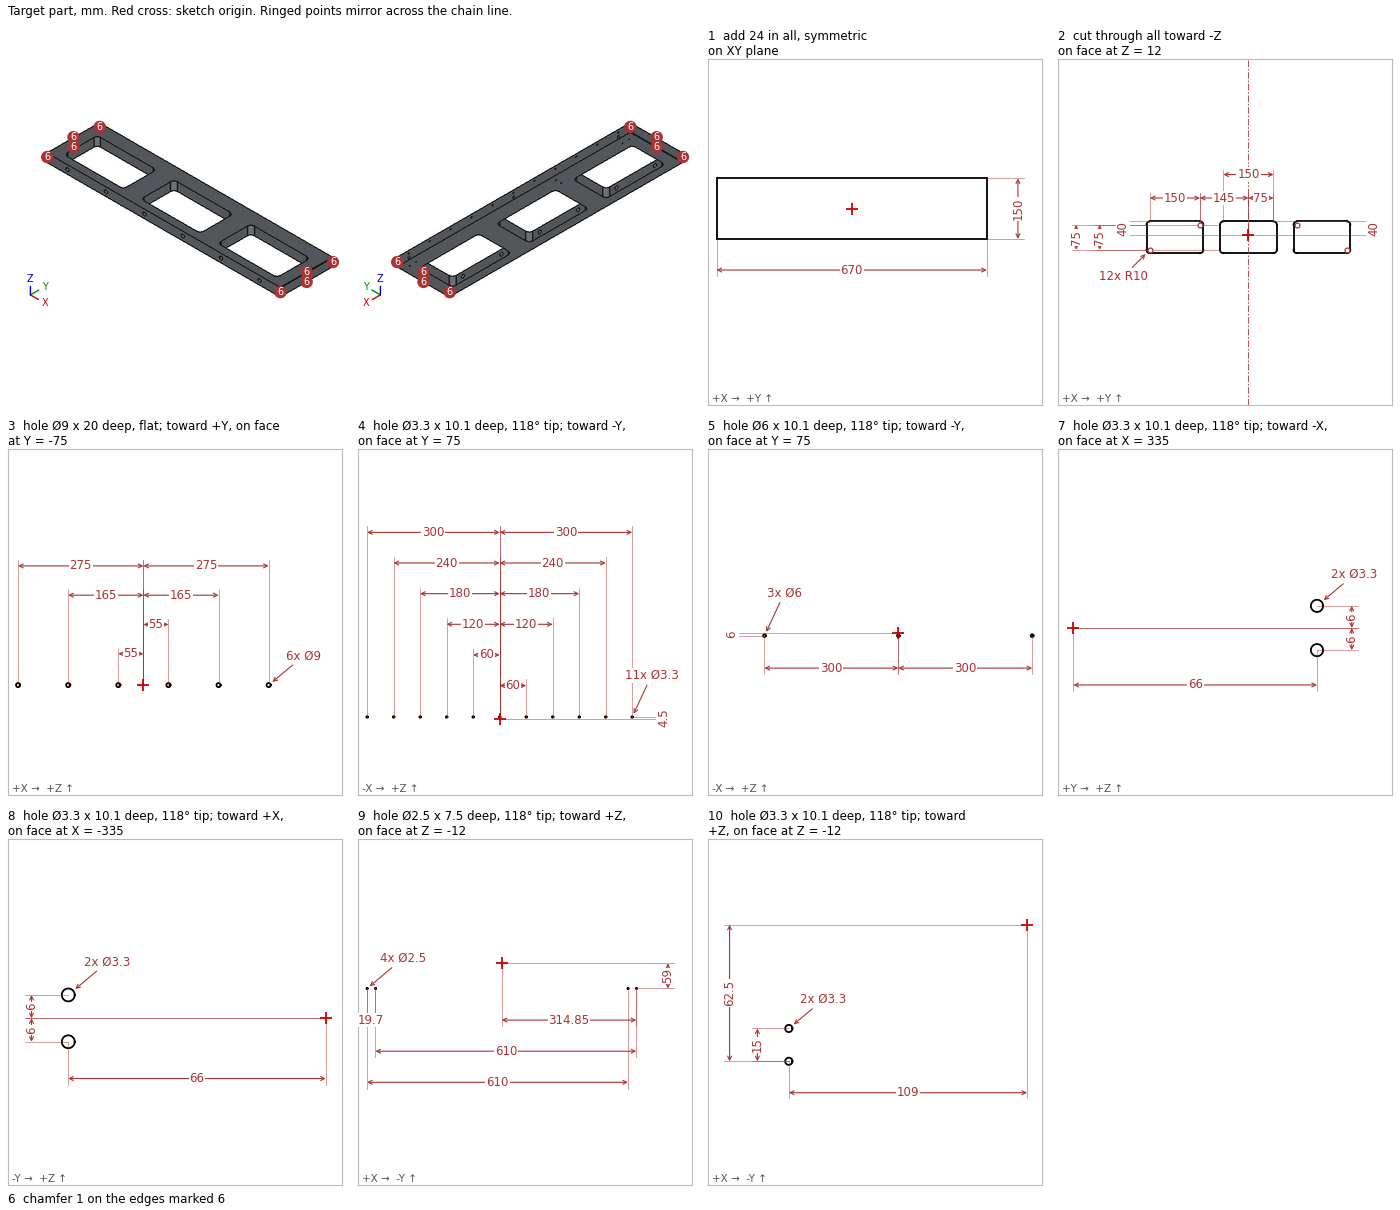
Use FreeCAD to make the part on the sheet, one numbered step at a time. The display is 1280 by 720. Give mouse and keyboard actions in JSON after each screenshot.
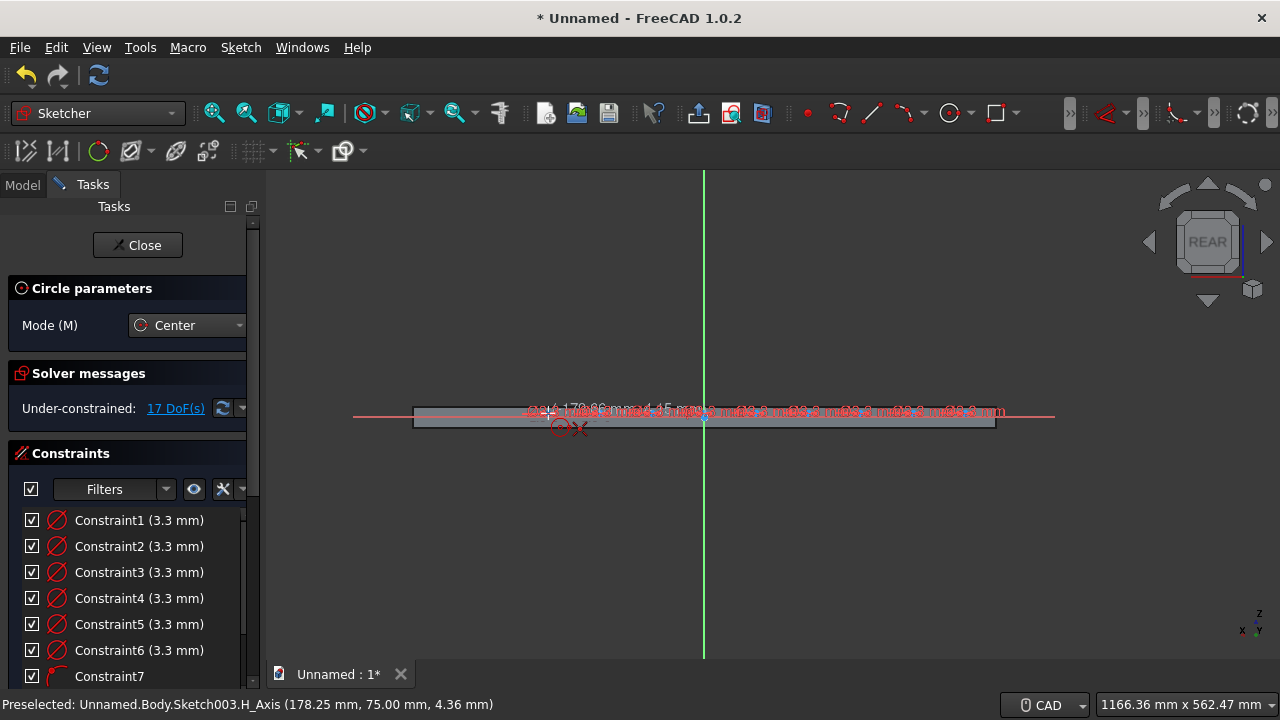
{"action": "scroll", "coordinate": [496, 413], "scroll_direction": "up", "scroll_amount": 14}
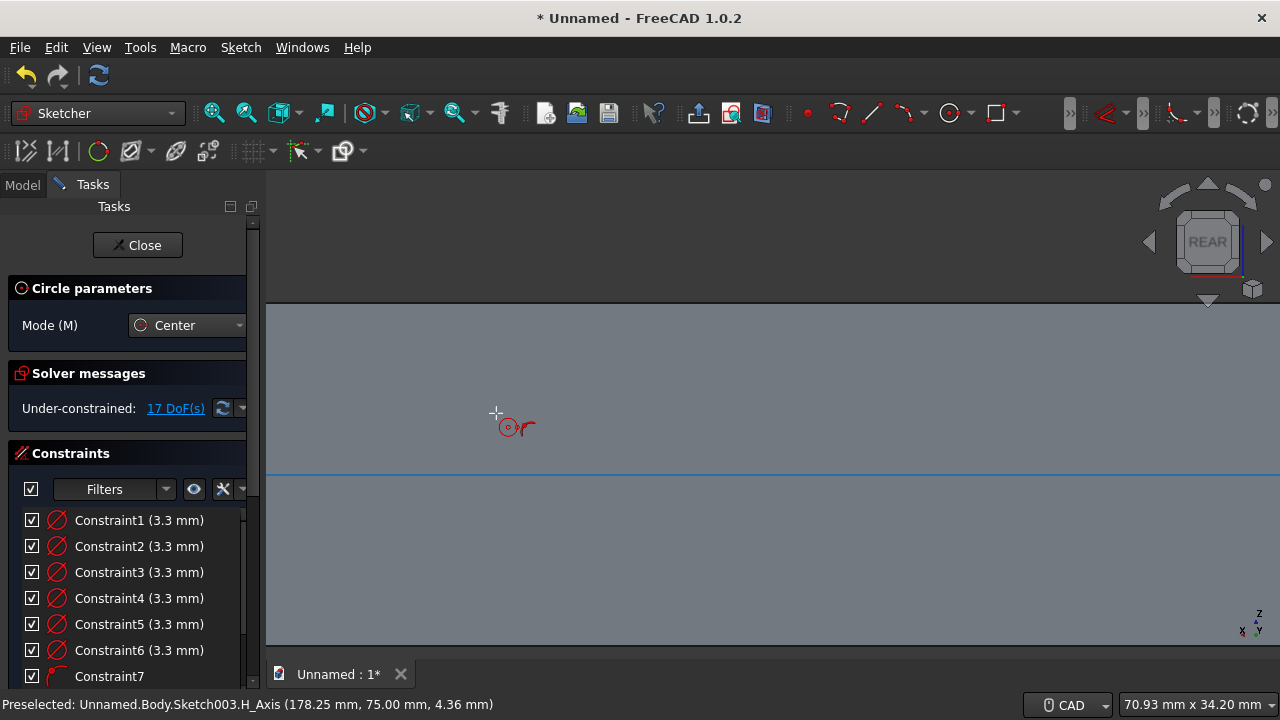
{"action": "scroll", "coordinate": [496, 413], "scroll_direction": "down", "scroll_amount": 14}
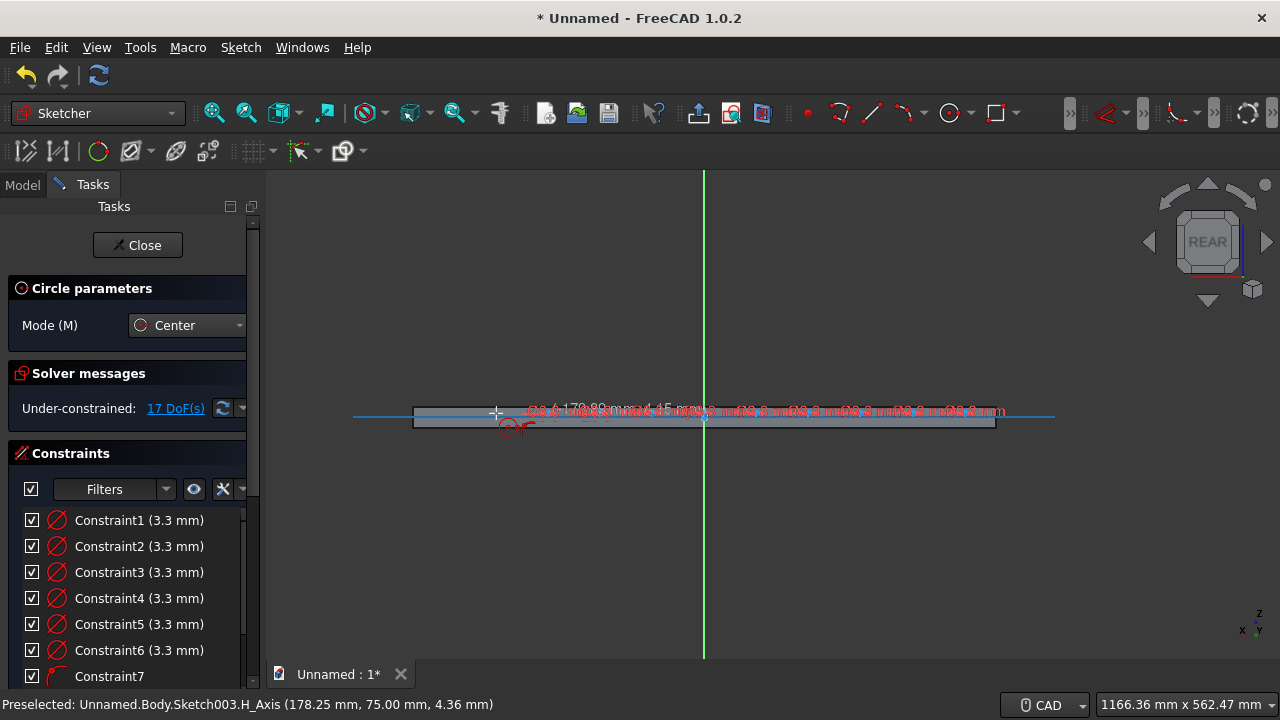
{"action": "scroll", "coordinate": [496, 413], "scroll_direction": "up", "scroll_amount": 8}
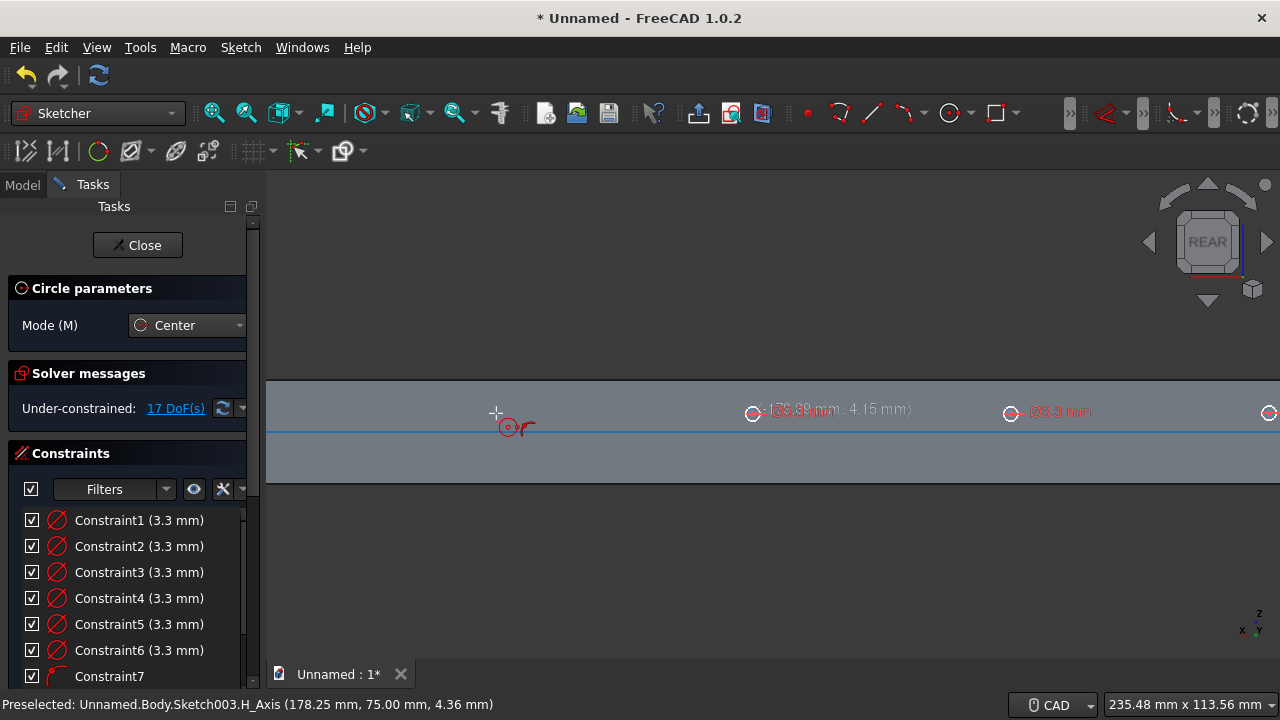
{"action": "left_click", "coordinate": [494, 413]}
{"action": "mouse_move", "coordinate": [499, 407]}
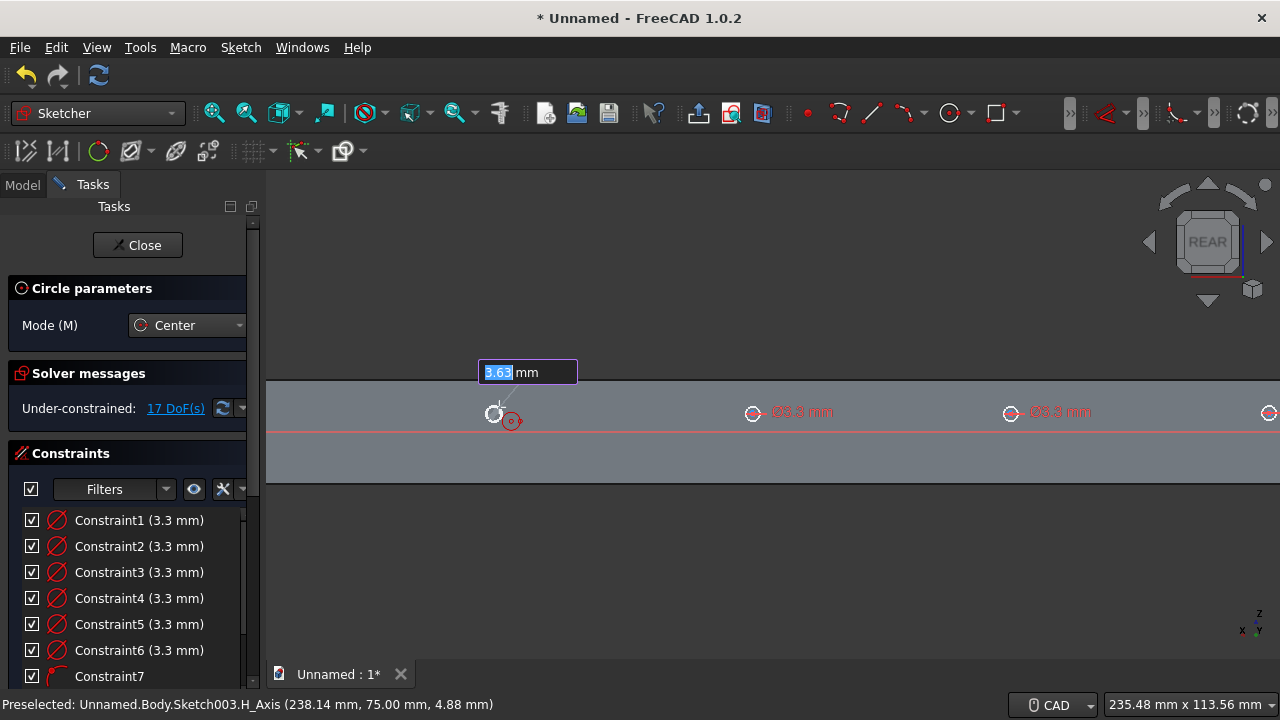
{"action": "type", "text": "3.3"}
{"action": "key", "text": "Return"}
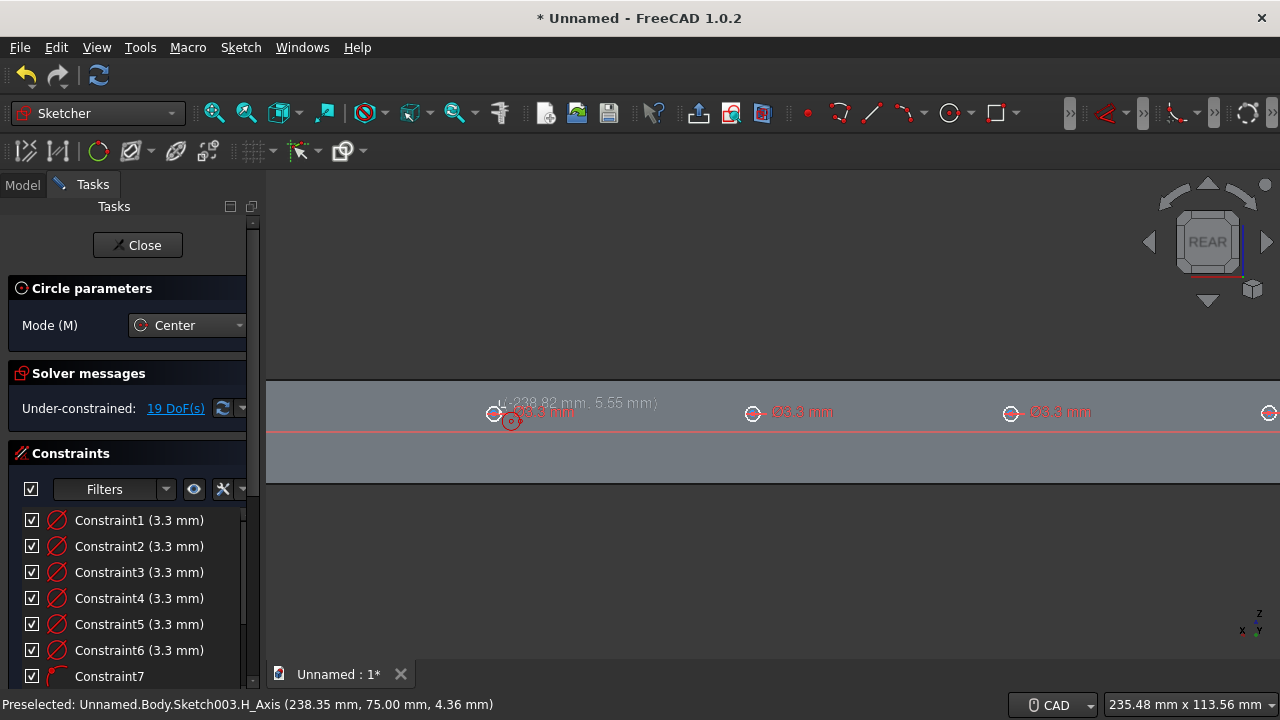
{"action": "scroll", "coordinate": [496, 413], "scroll_direction": "down", "scroll_amount": 8}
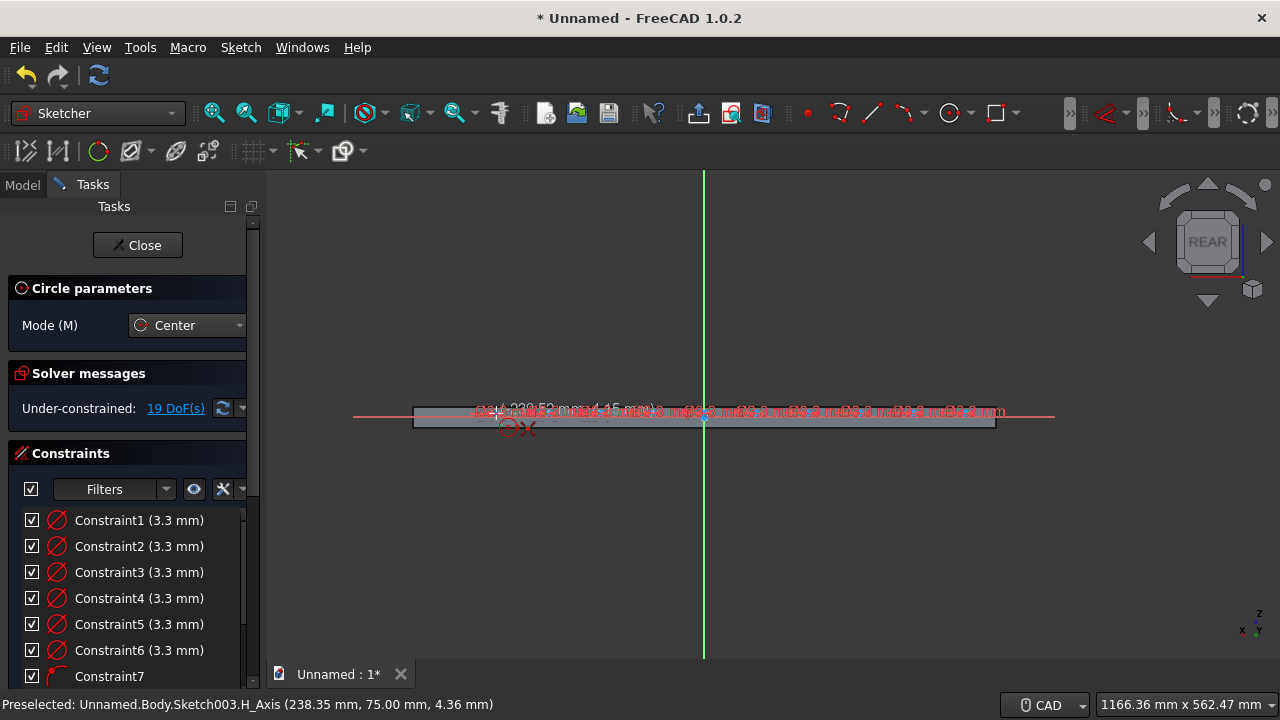
{"action": "scroll", "coordinate": [444, 413], "scroll_direction": "up", "scroll_amount": 14}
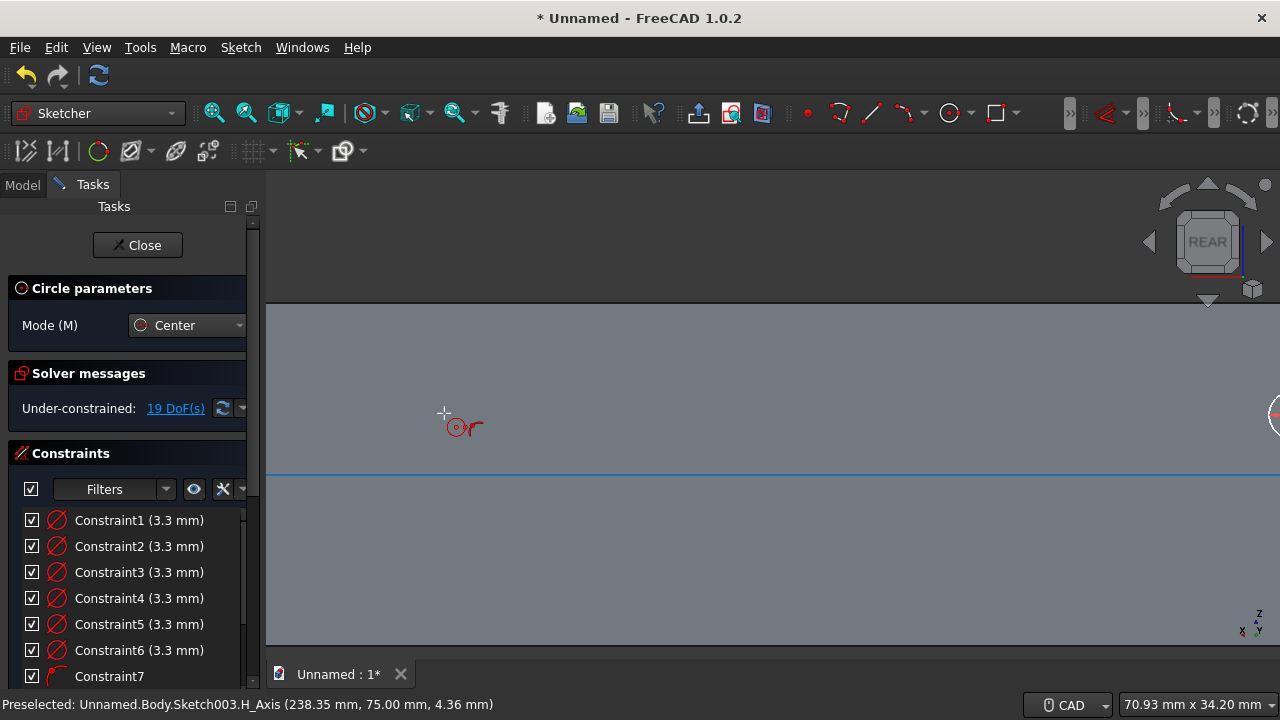
{"action": "scroll", "coordinate": [444, 413], "scroll_direction": "down", "scroll_amount": 14}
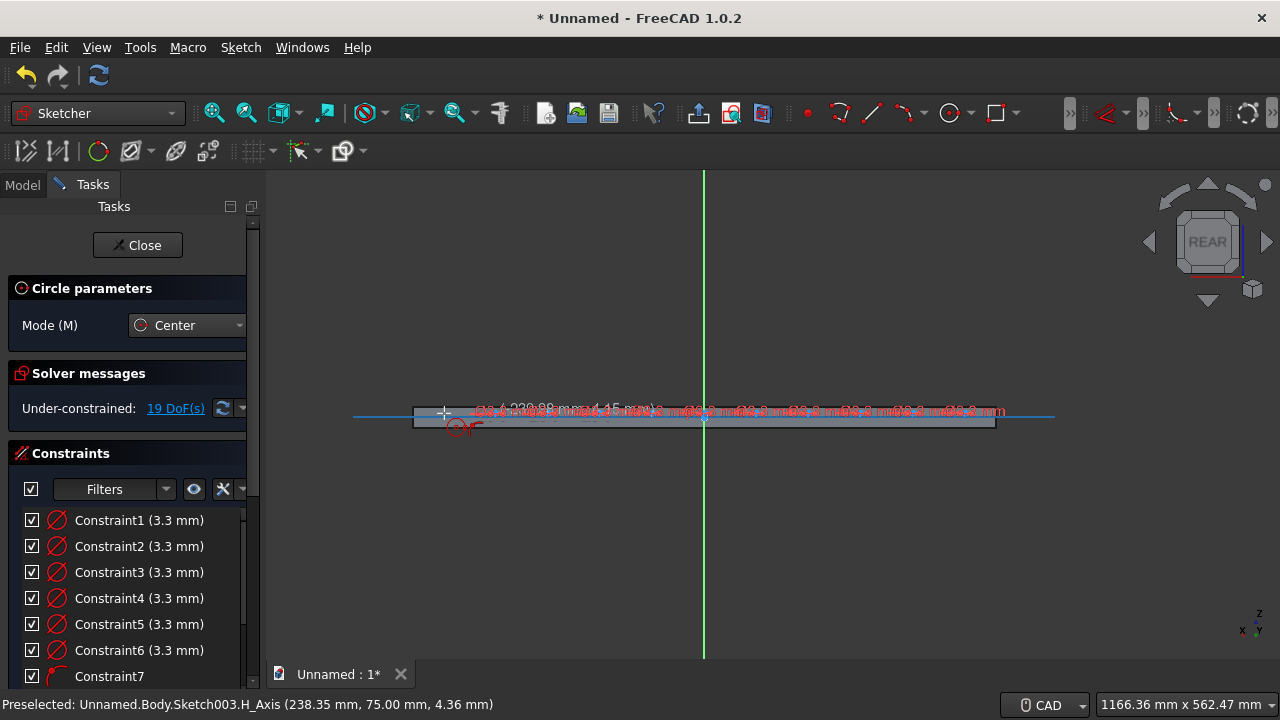
{"action": "scroll", "coordinate": [444, 413], "scroll_direction": "up", "scroll_amount": 8}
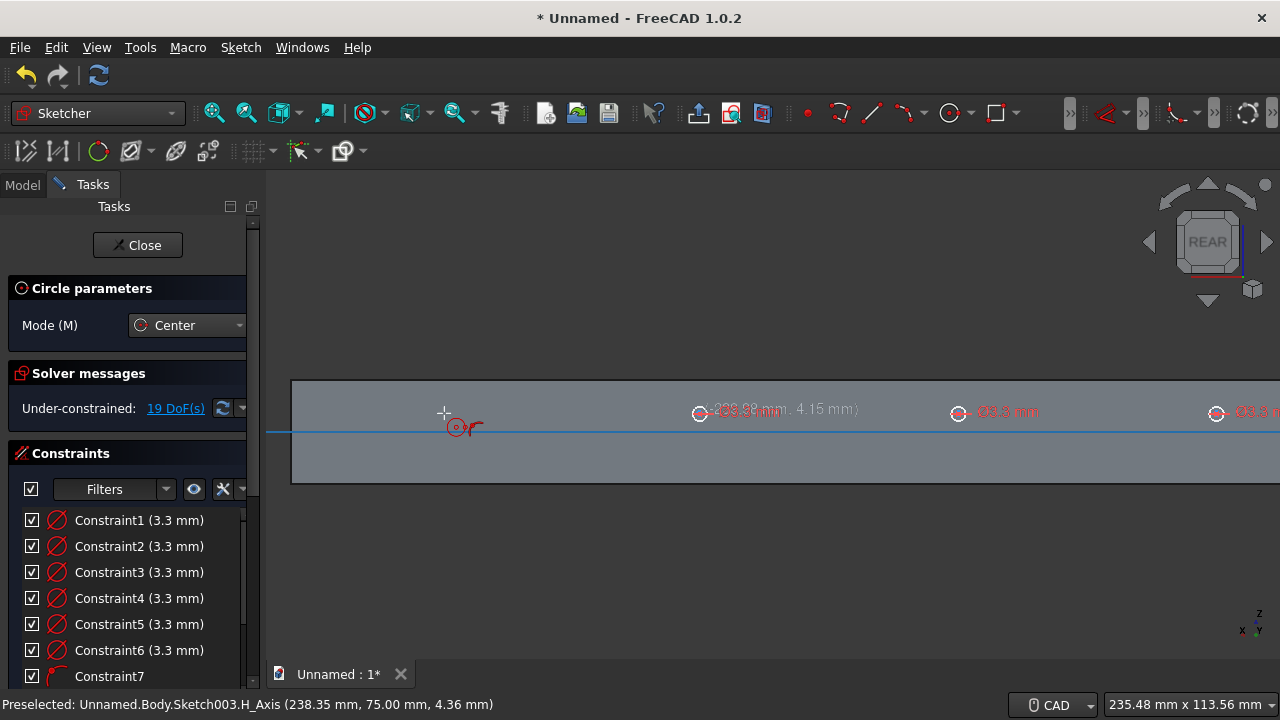
{"action": "left_click", "coordinate": [441, 413]}
{"action": "mouse_move", "coordinate": [446, 407]}